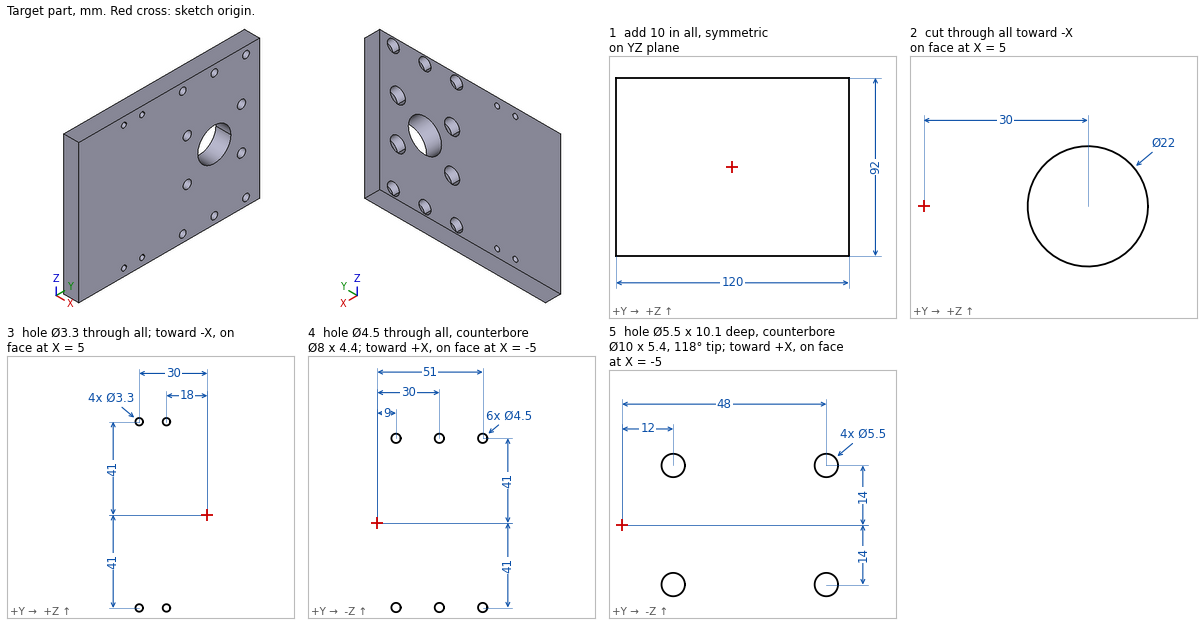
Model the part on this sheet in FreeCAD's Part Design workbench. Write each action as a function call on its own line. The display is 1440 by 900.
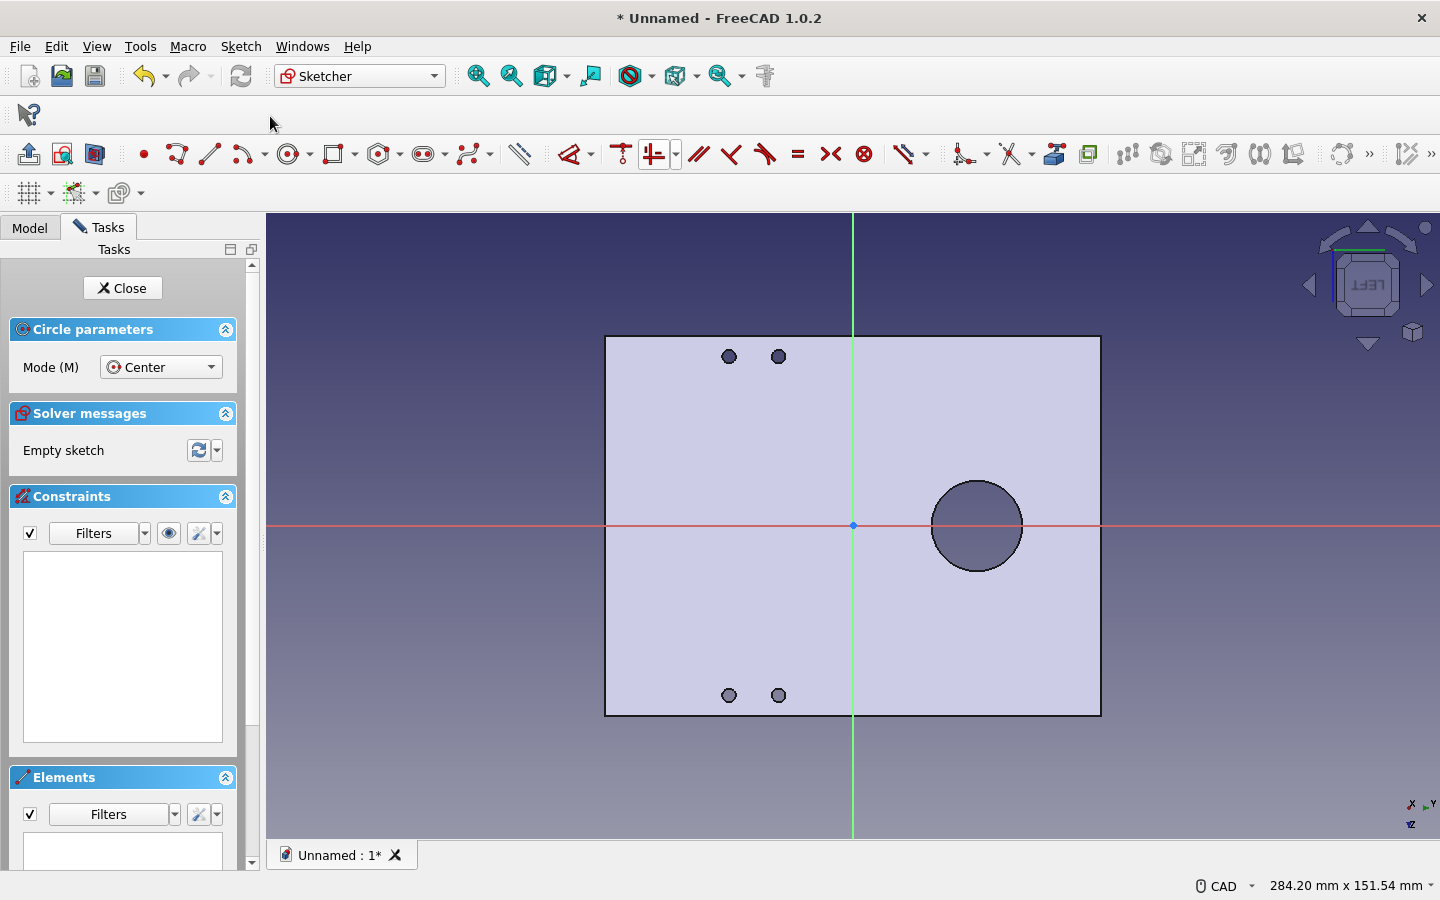
scroll(1064, 357, up, 5)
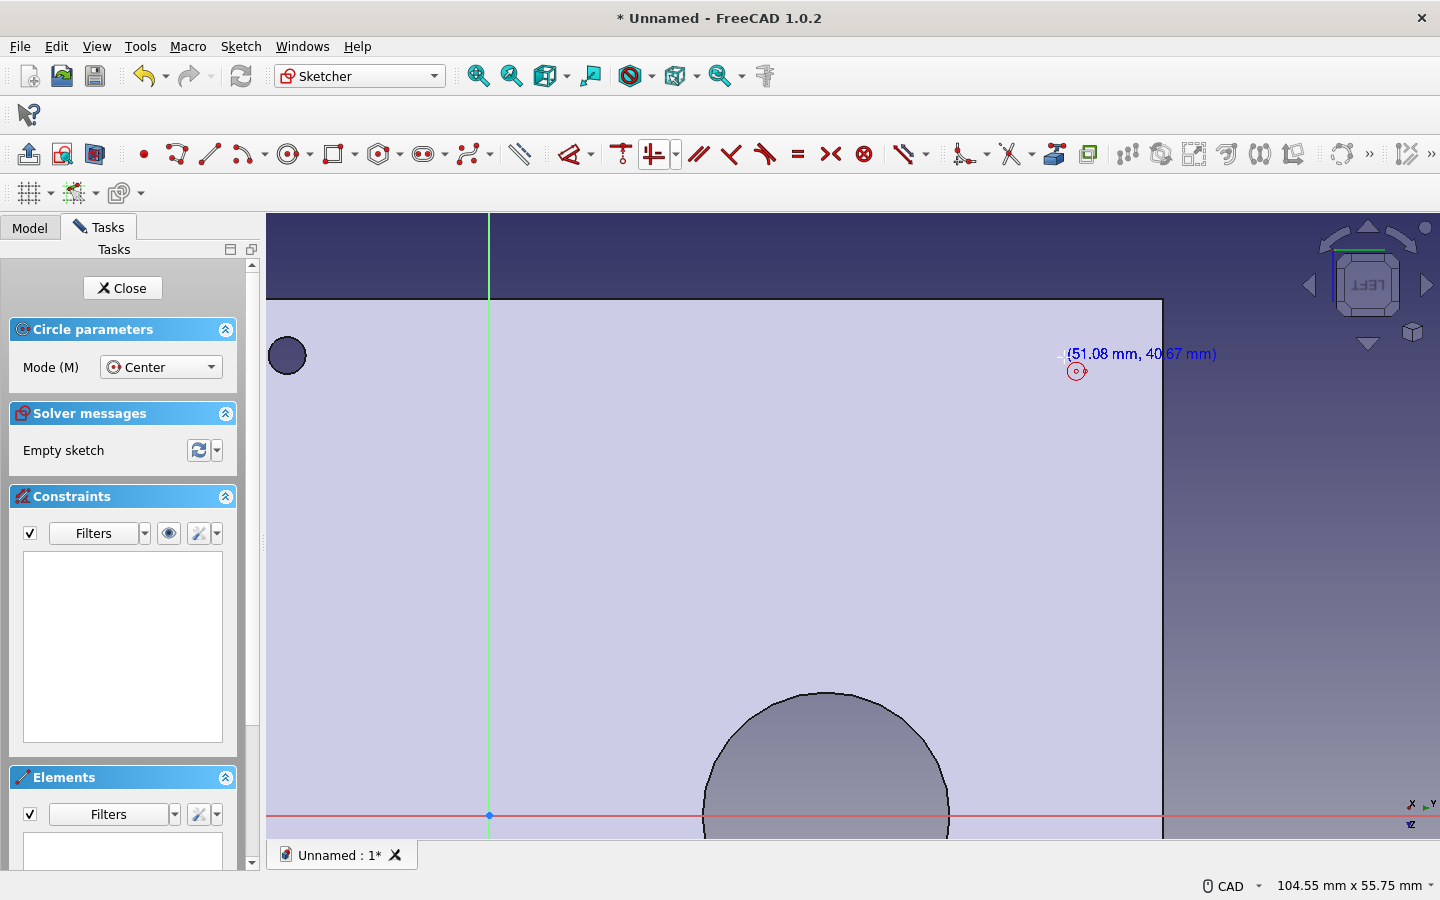
click(1062, 356)
click(1080, 338)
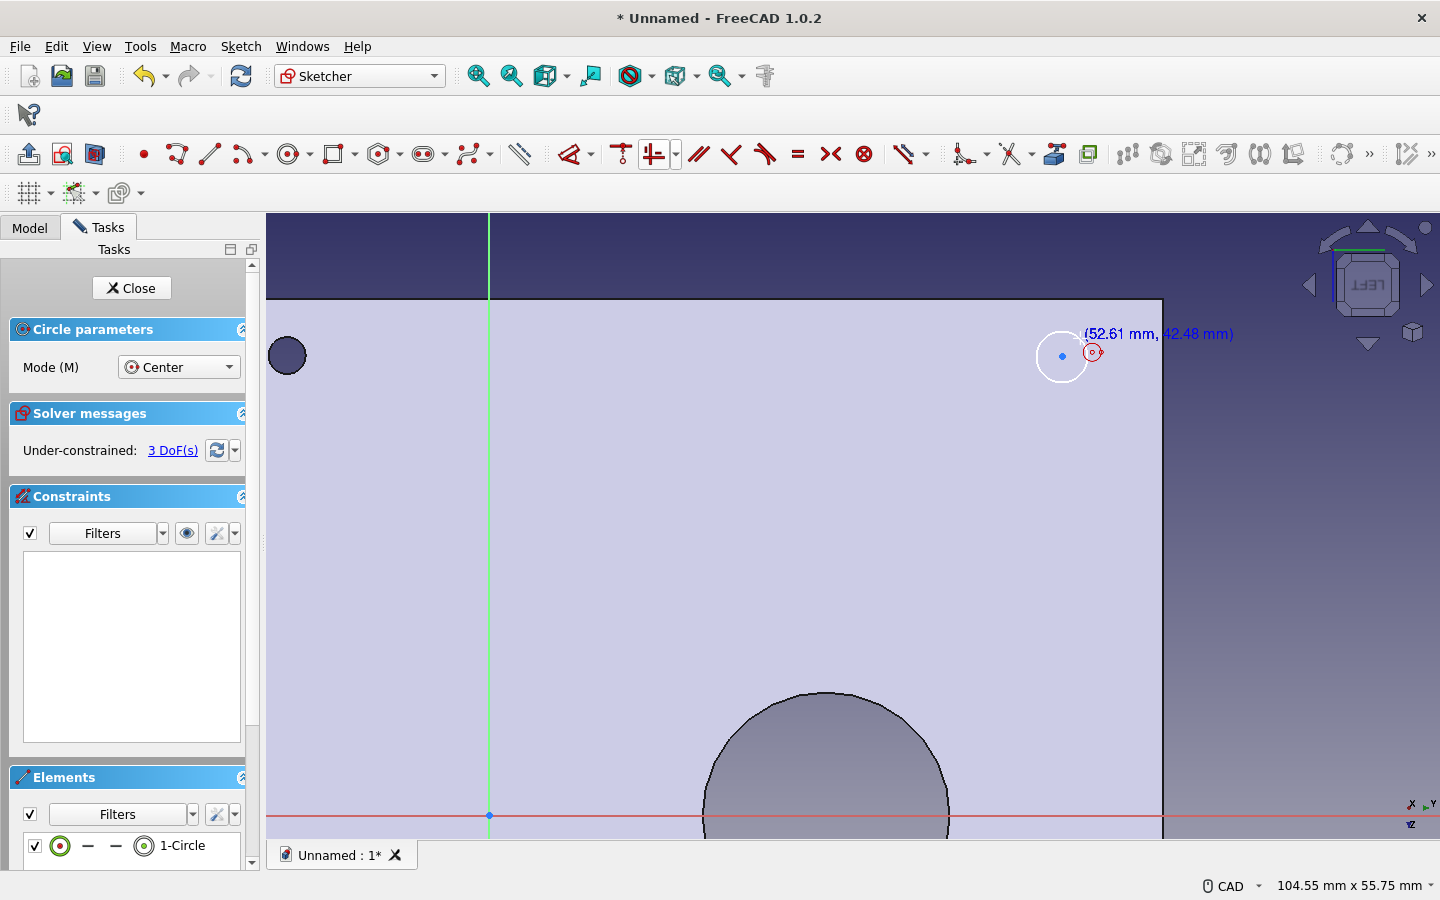
click(826, 356)
click(844, 338)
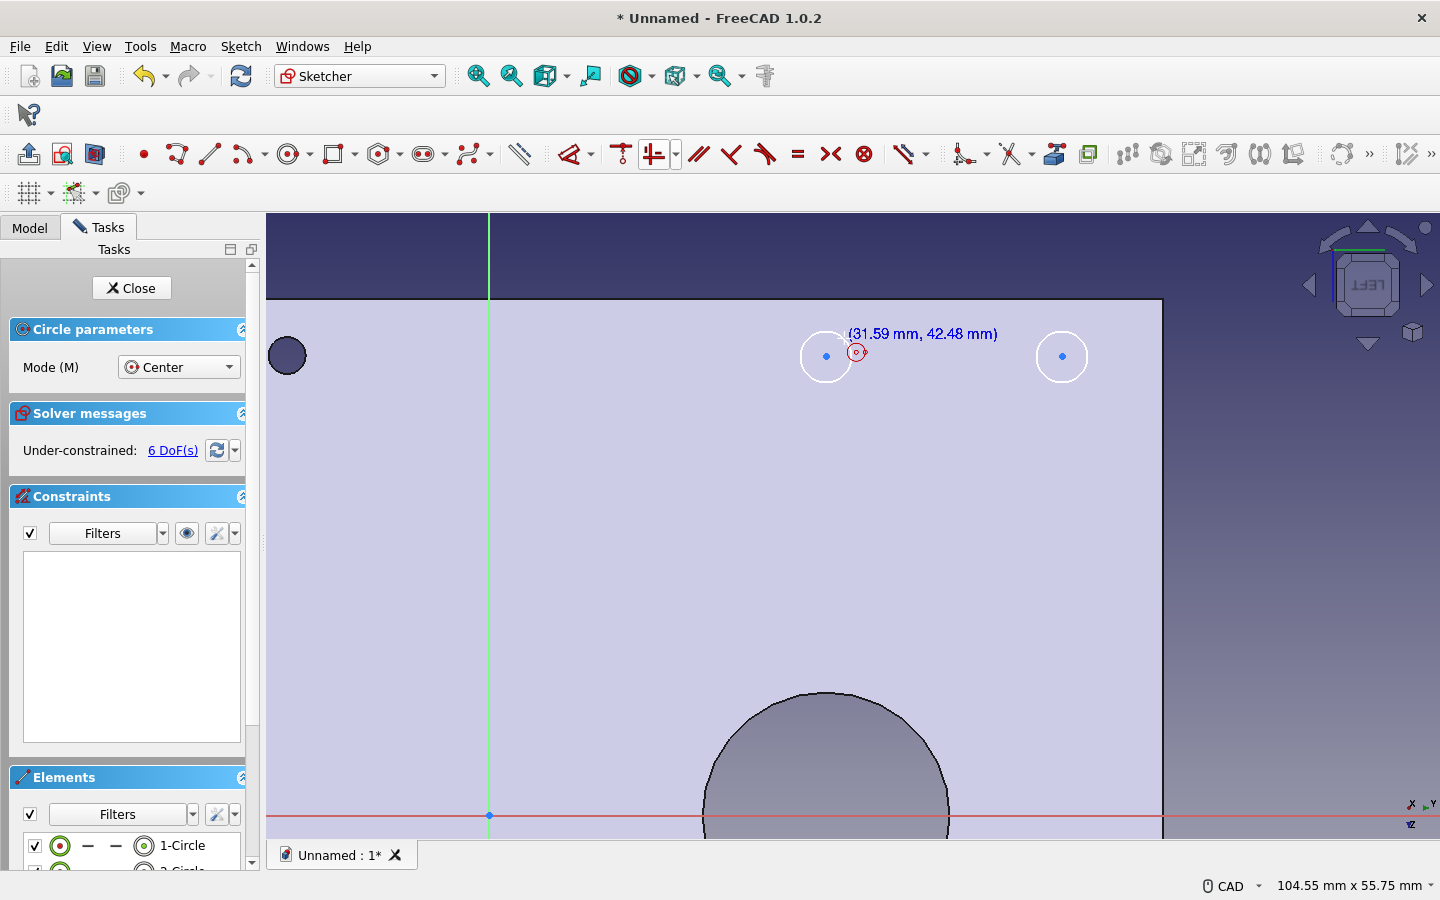
click(590, 356)
click(608, 338)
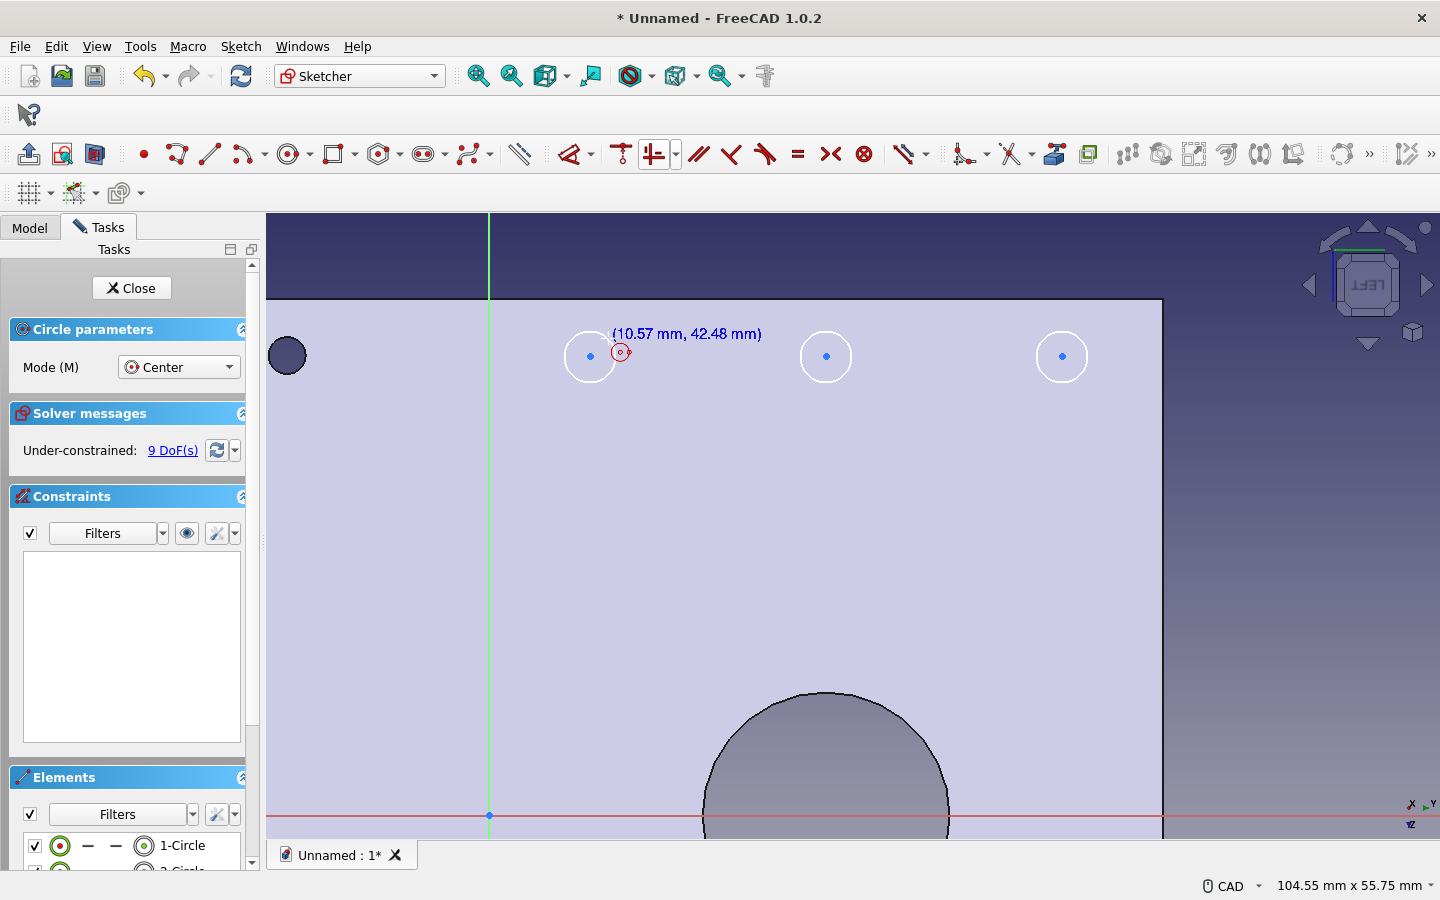
scroll(781, 289, down, 4)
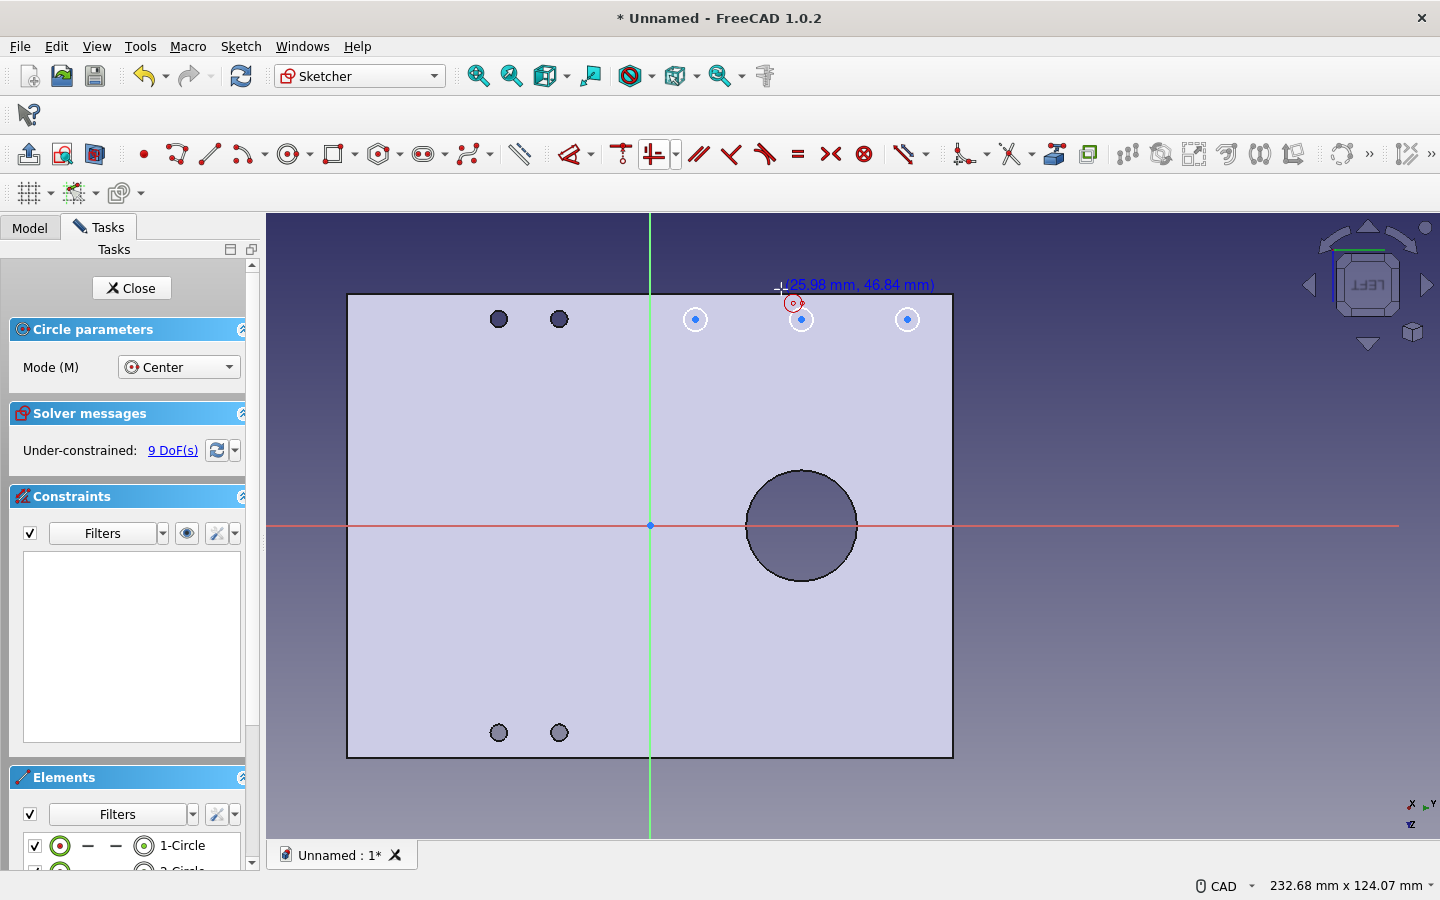
scroll(907, 733, up, 4)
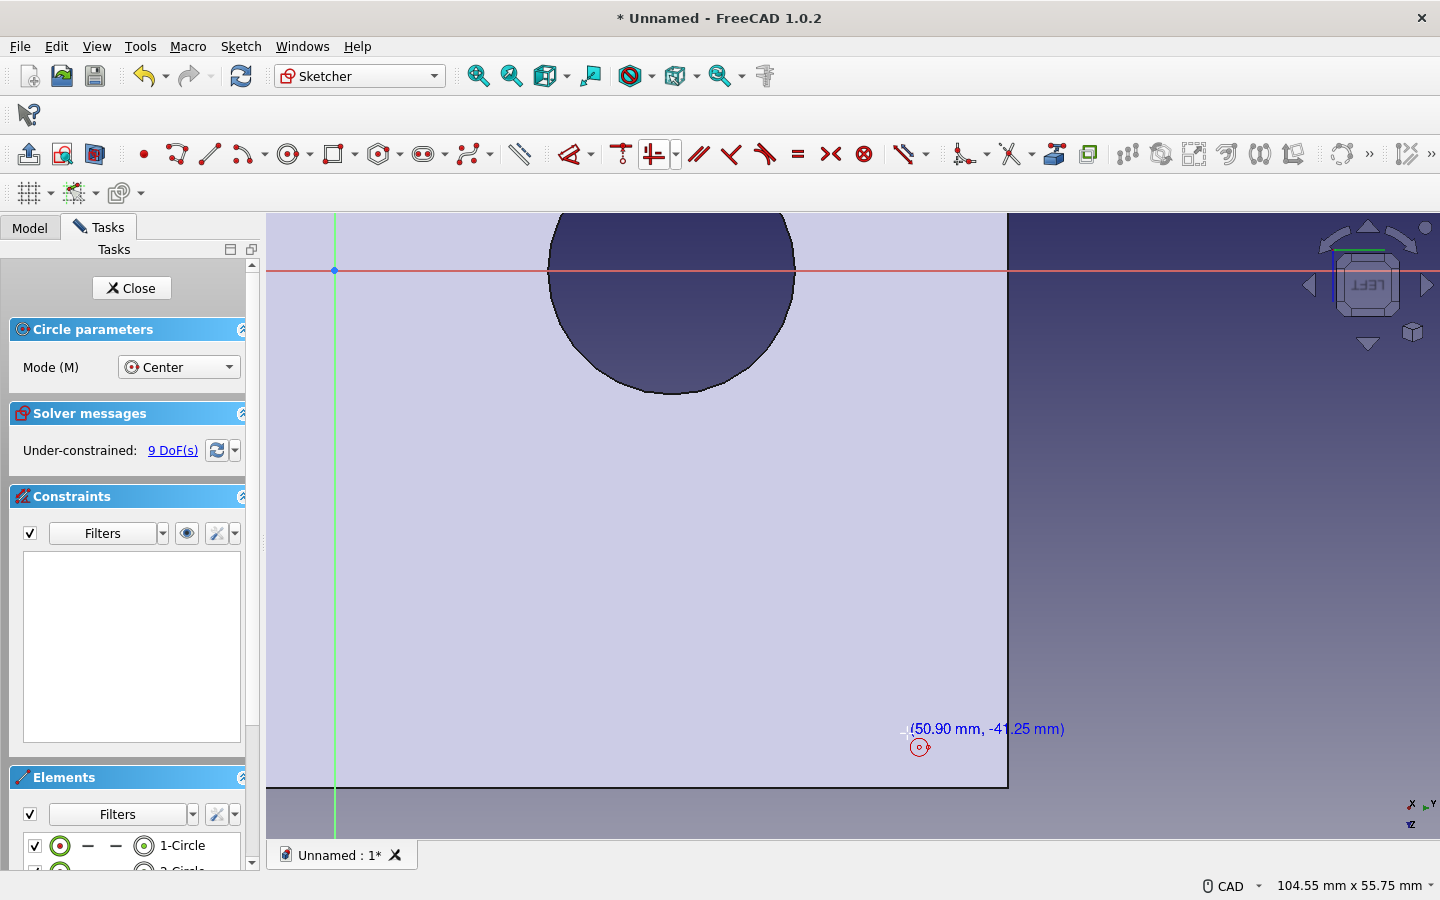
click(907, 731)
click(925, 714)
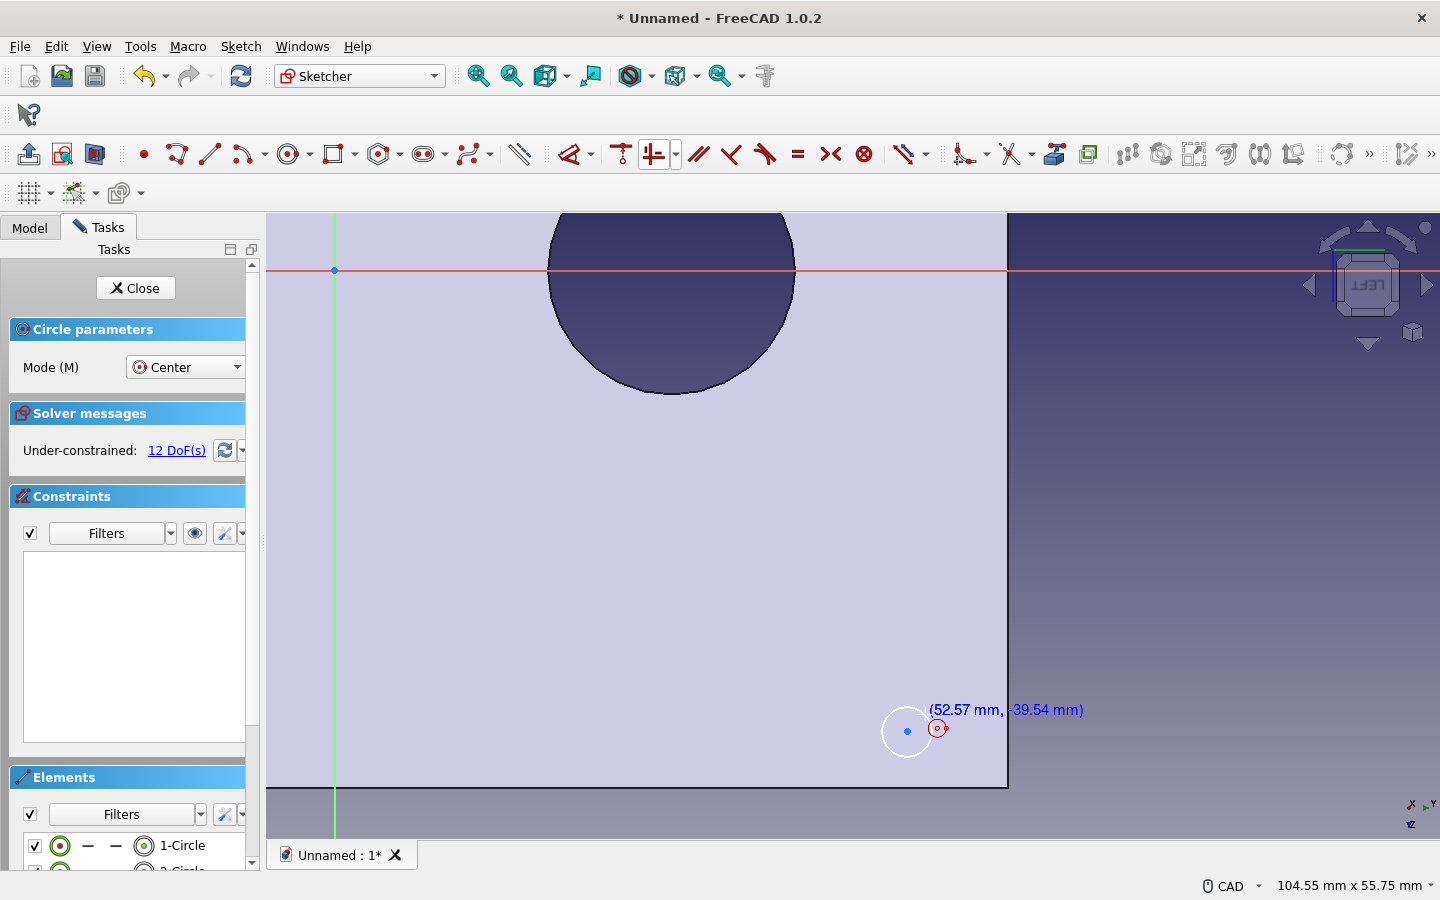
click(672, 731)
click(689, 714)